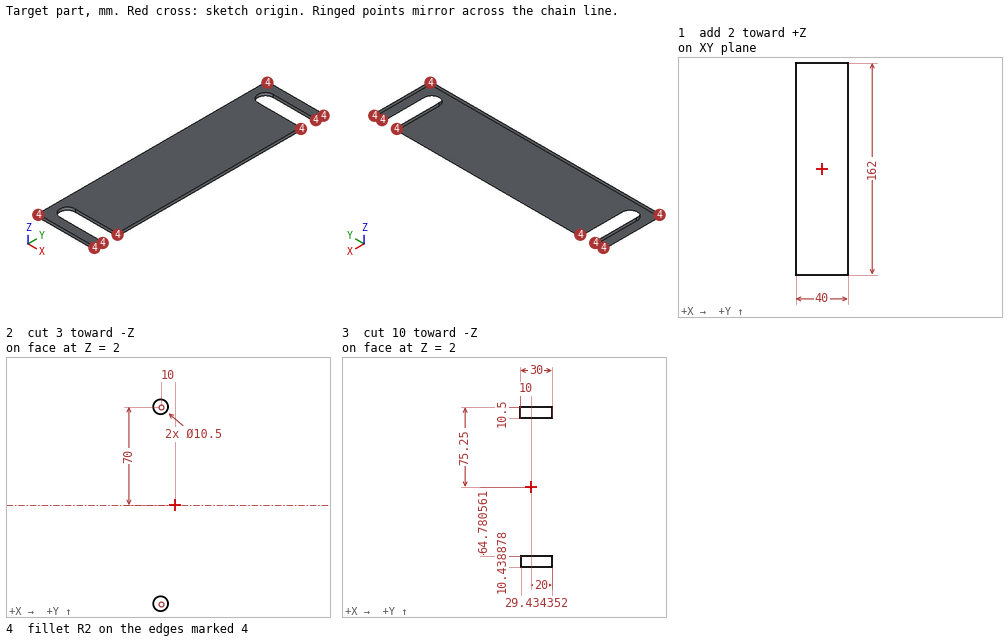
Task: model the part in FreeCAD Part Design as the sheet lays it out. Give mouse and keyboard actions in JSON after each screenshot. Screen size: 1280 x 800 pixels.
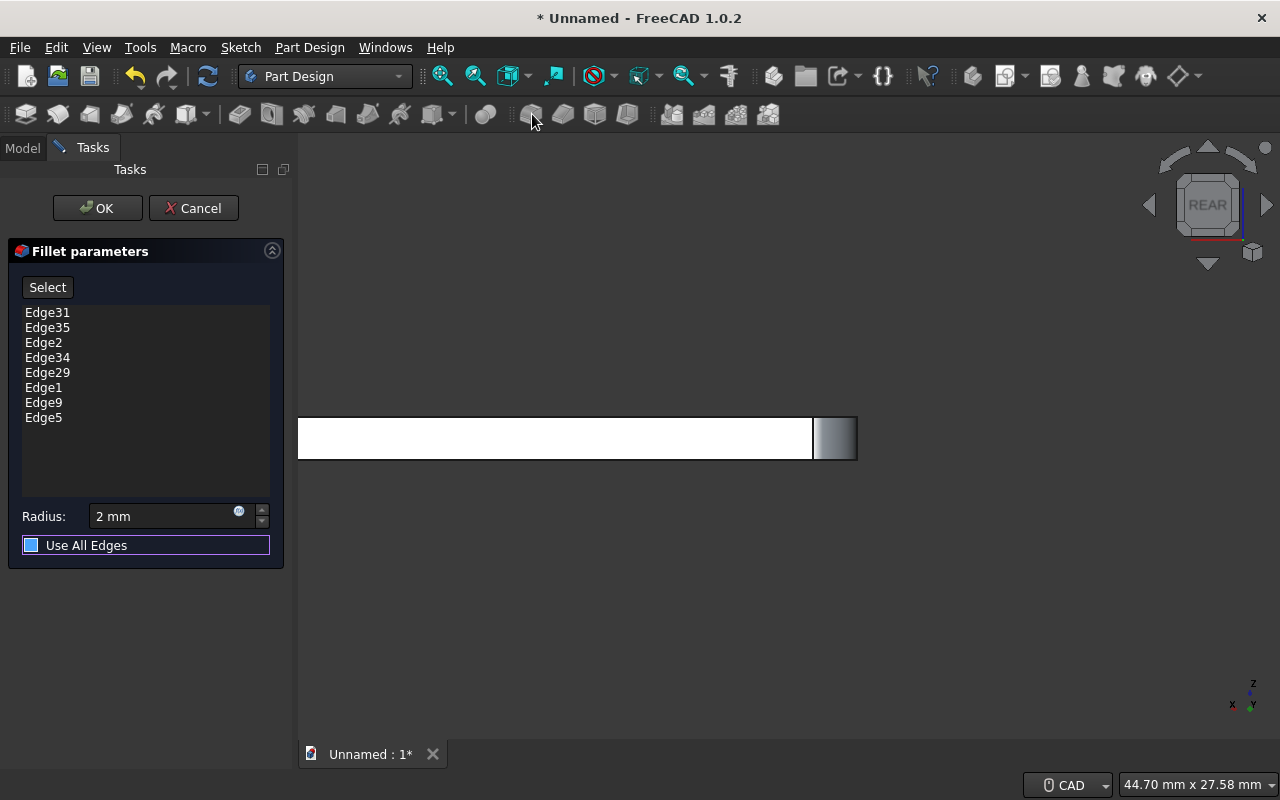
{"action": "left_click", "coordinate": [98, 208]}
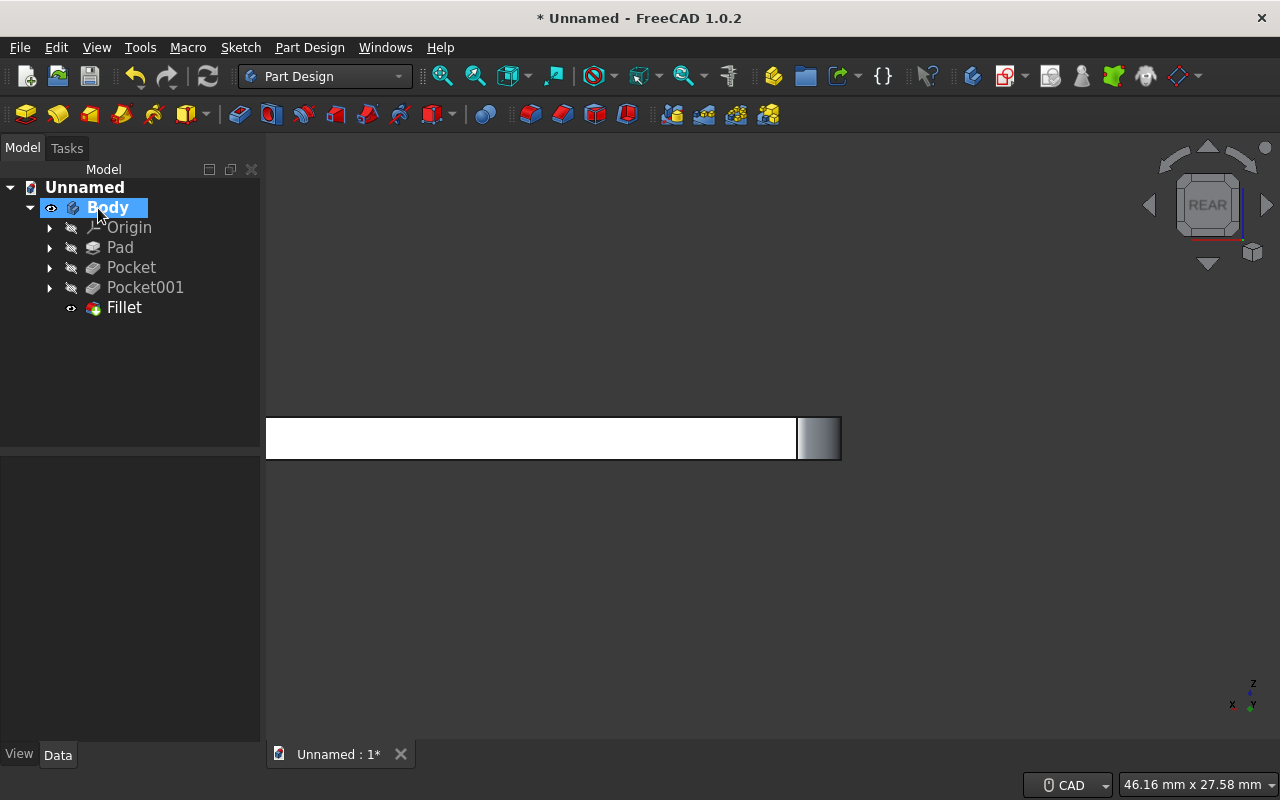
{"action": "key", "text": "0"}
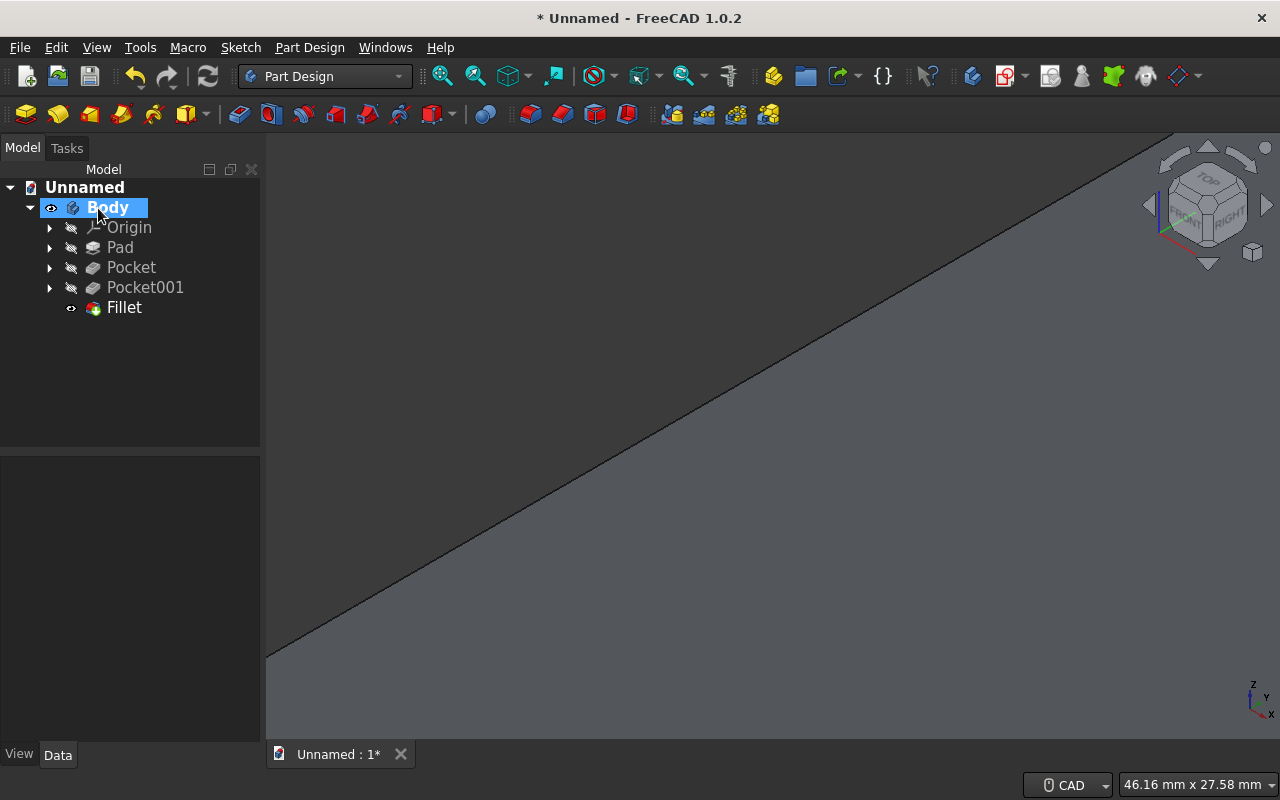
{"action": "left_click", "coordinate": [444, 76]}